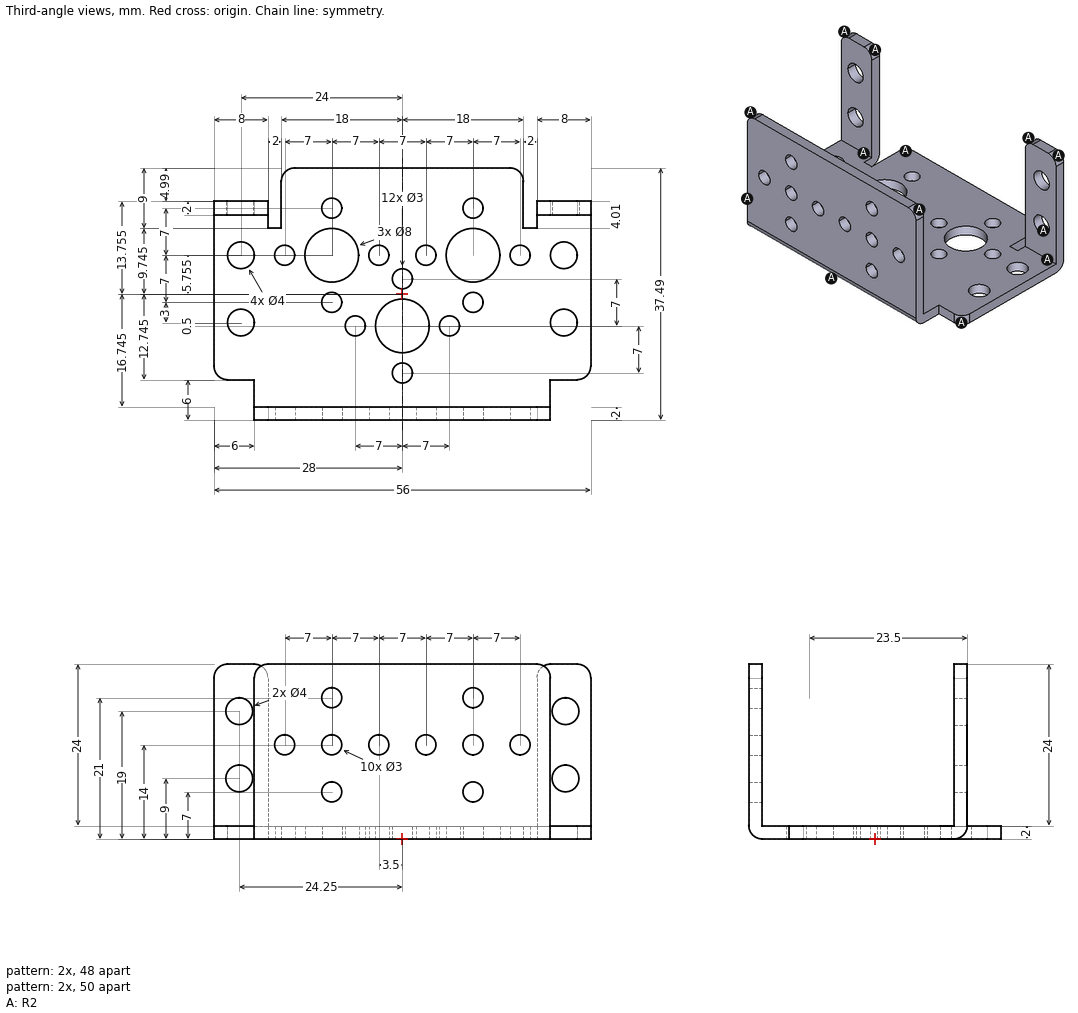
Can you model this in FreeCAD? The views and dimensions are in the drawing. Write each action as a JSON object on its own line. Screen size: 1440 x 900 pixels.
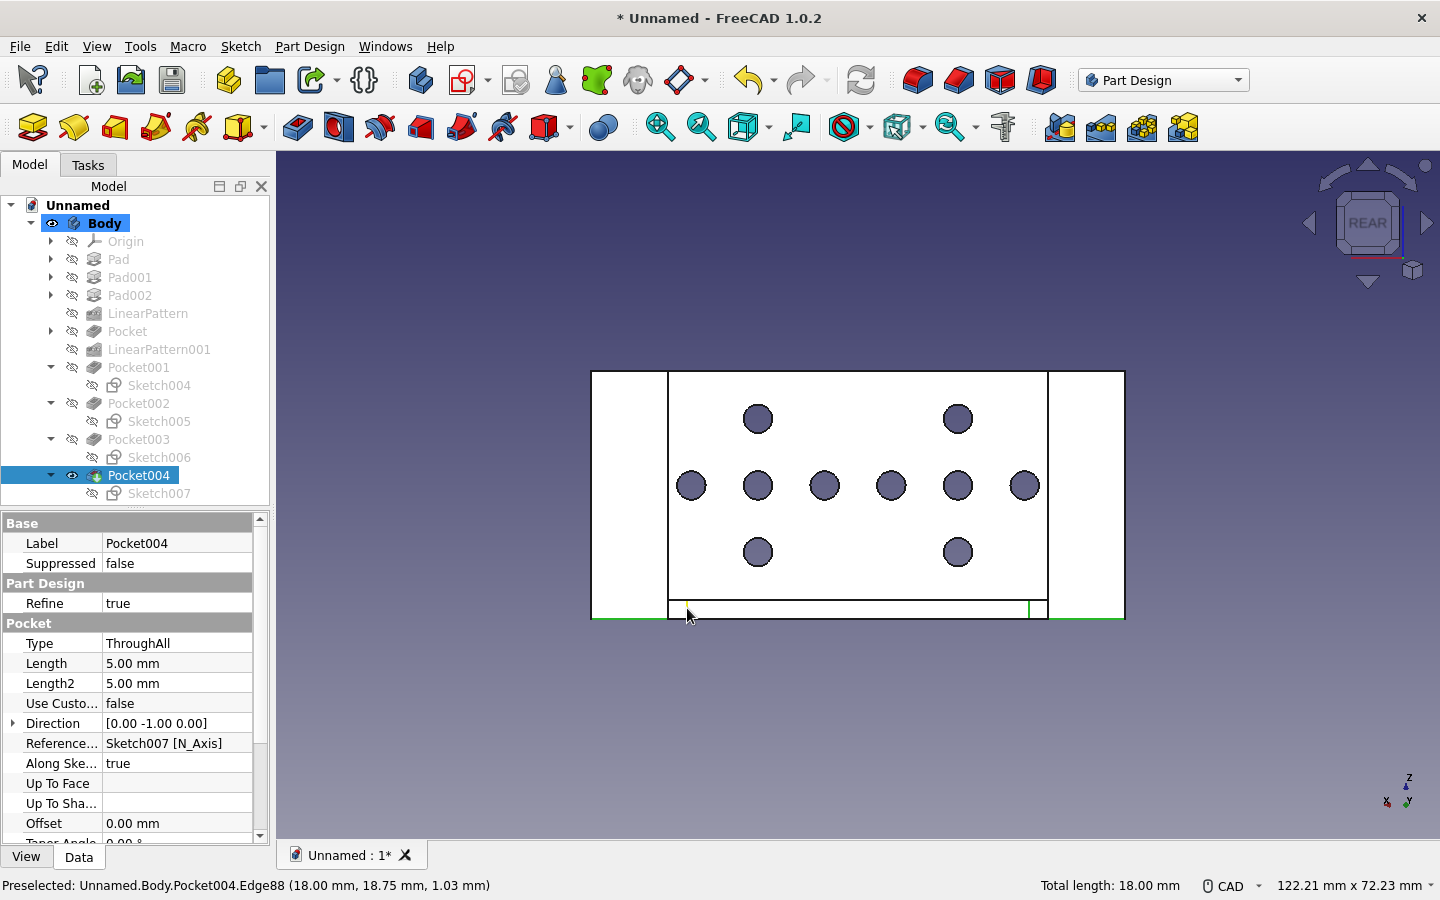
{"action": "key", "text": "0"}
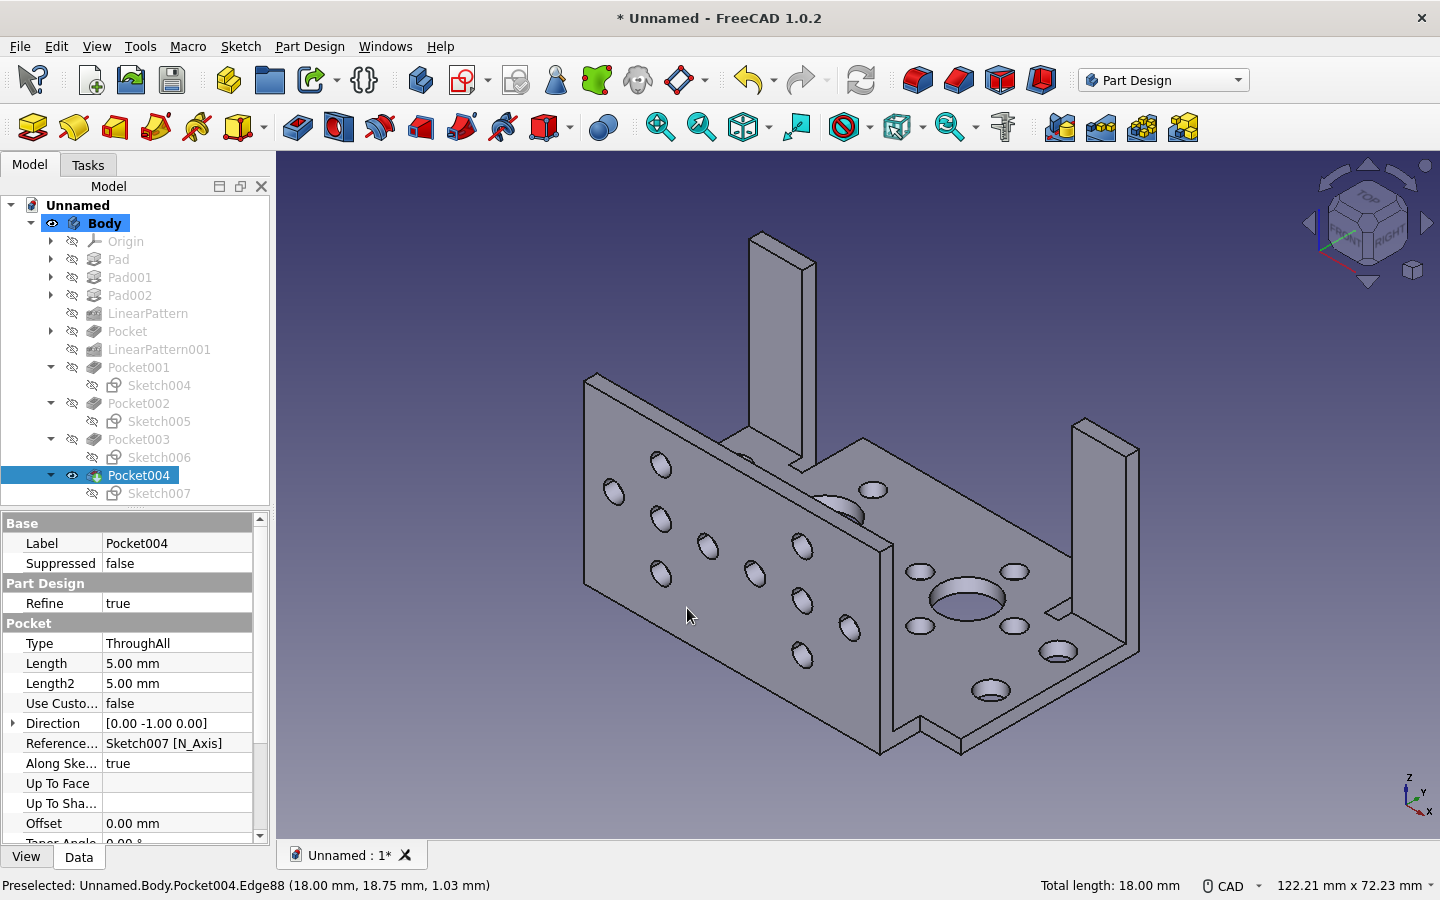
{"action": "left_click", "coordinate": [809, 266], "text": "ctrl"}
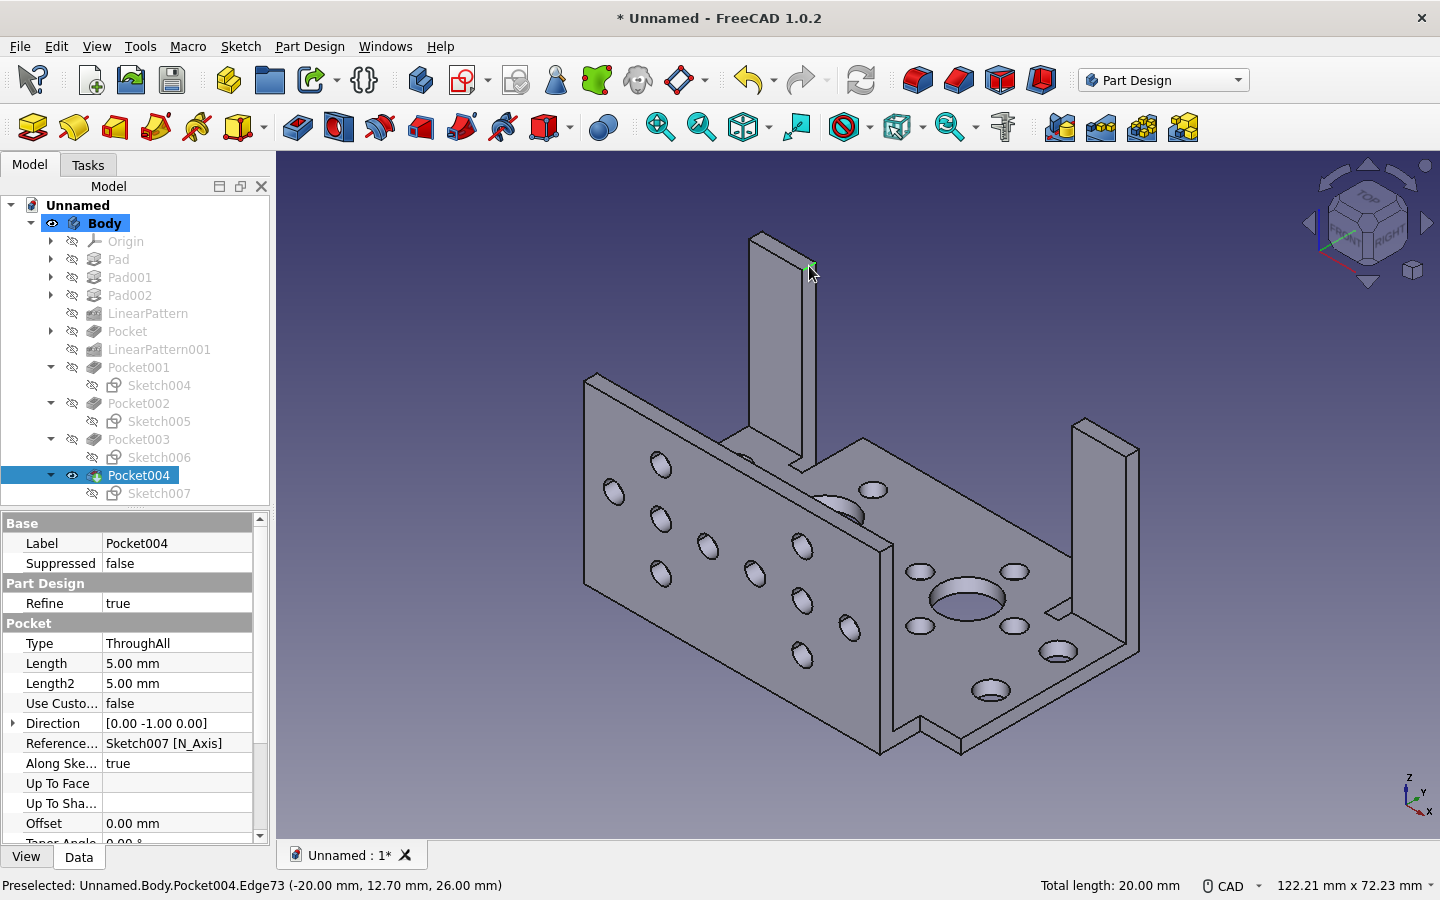
{"action": "left_click", "coordinate": [1132, 452], "text": "ctrl"}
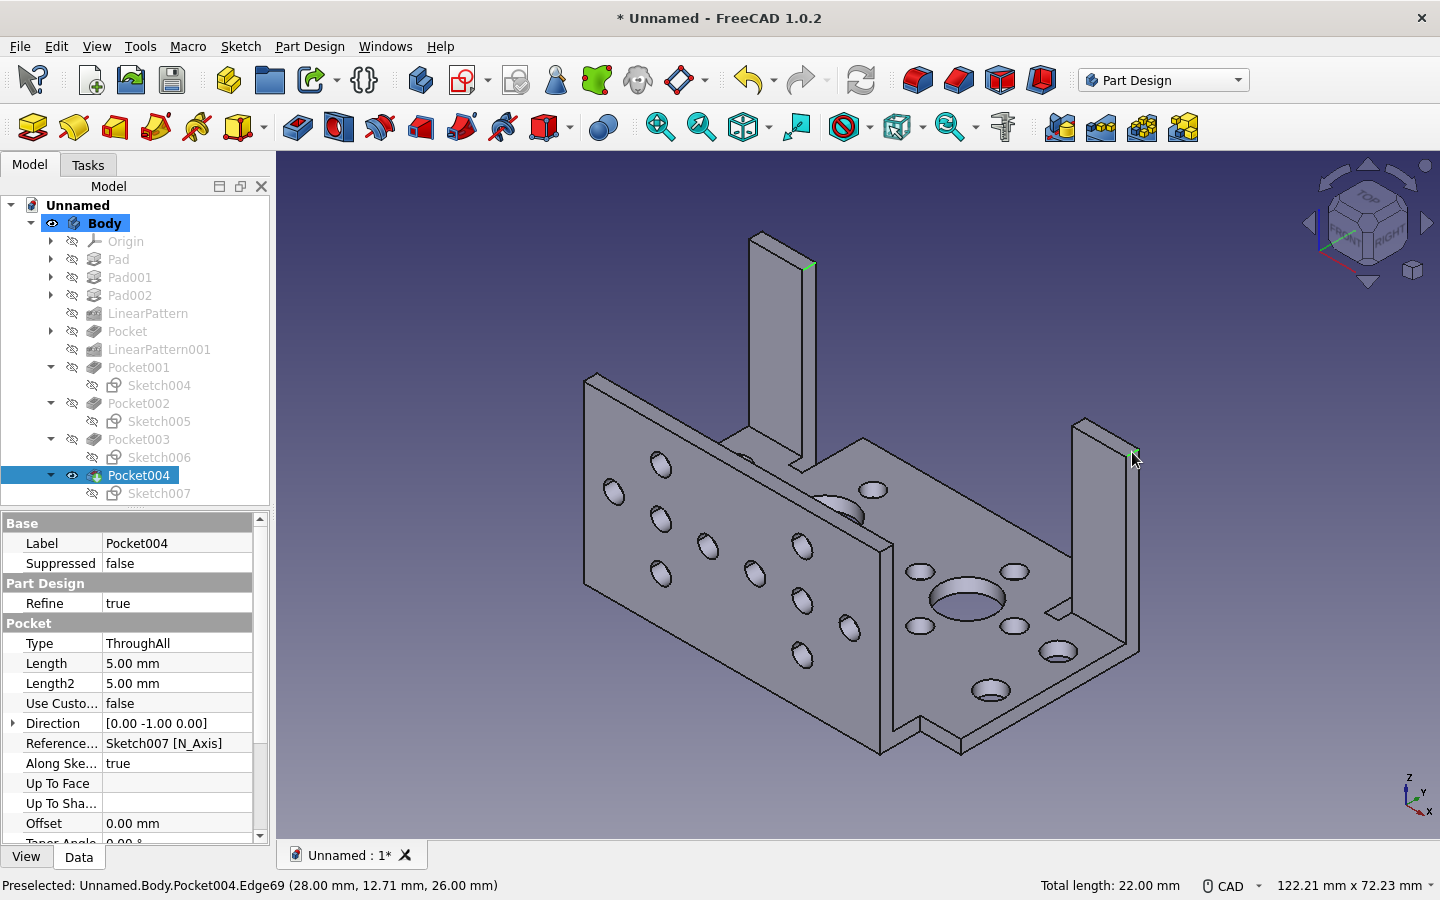
{"action": "left_click", "coordinate": [887, 547], "text": "ctrl"}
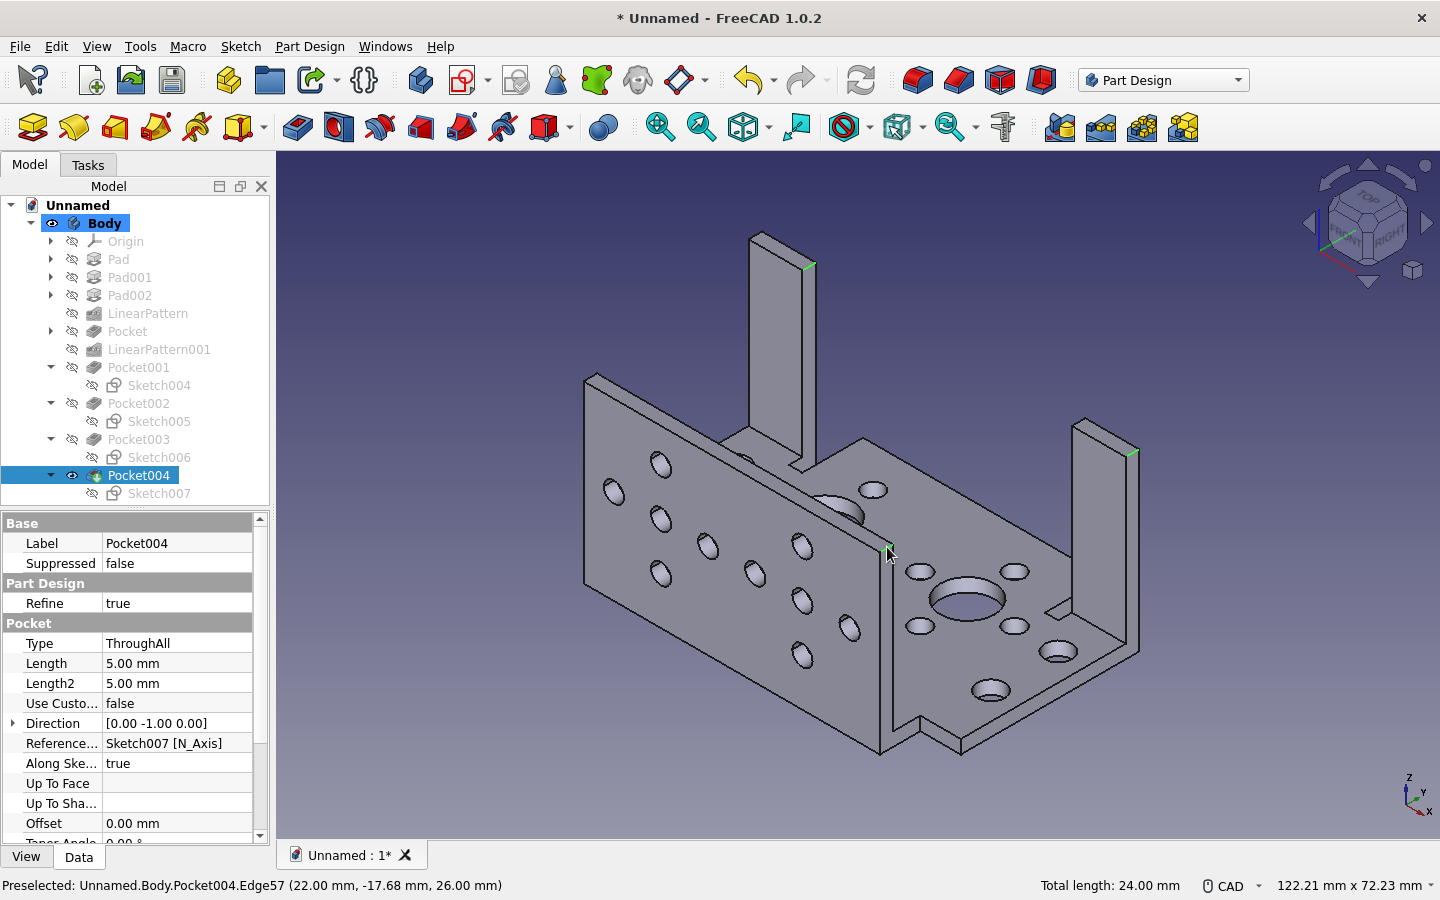
{"action": "left_click", "coordinate": [961, 746], "text": "ctrl"}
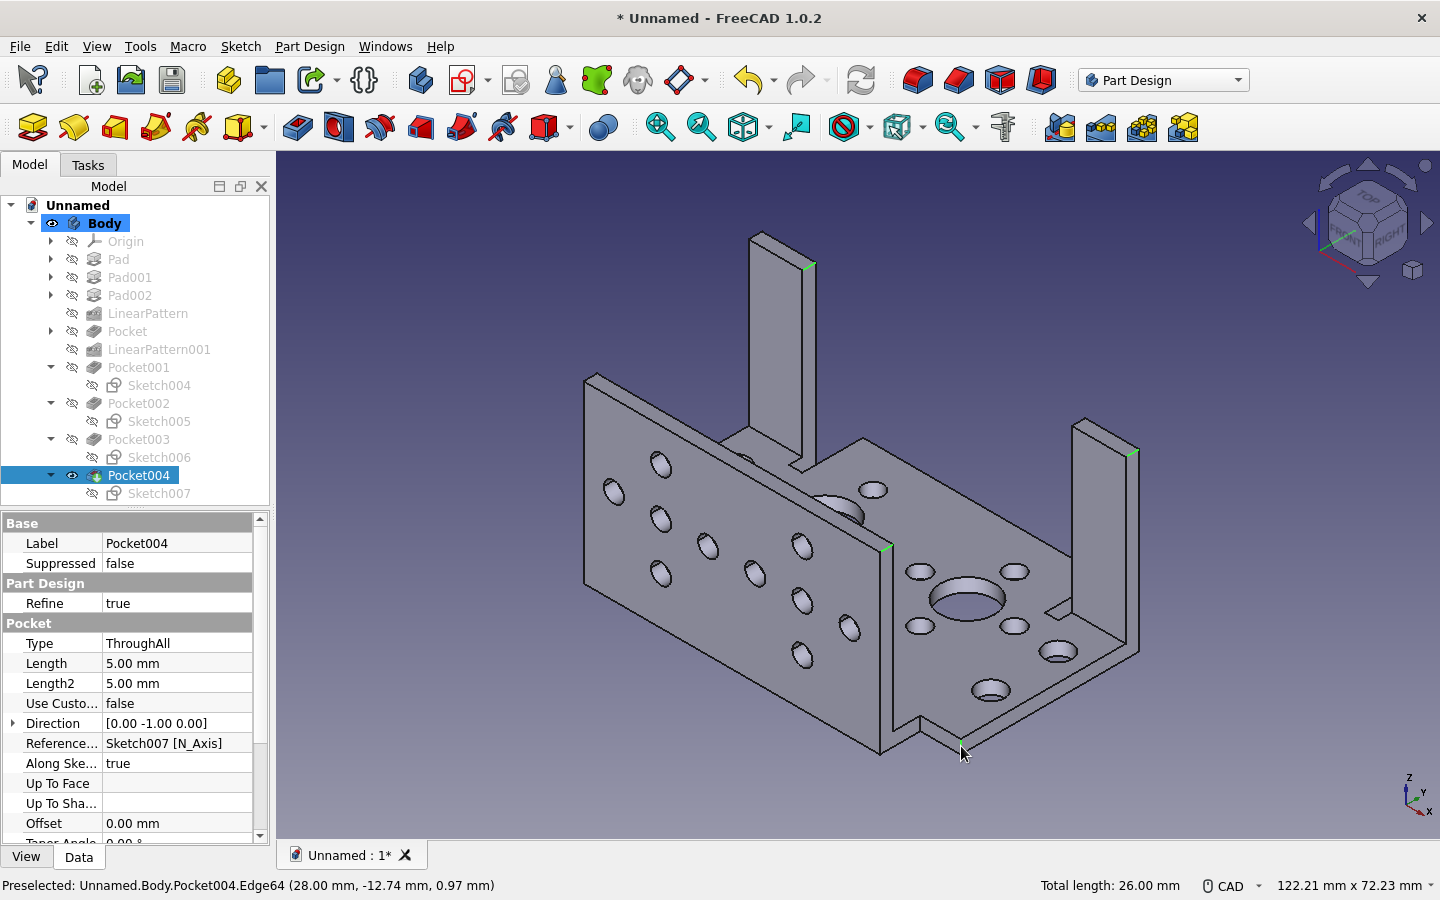
{"action": "scroll", "coordinate": [1105, 584], "scroll_direction": "up", "scroll_amount": 4}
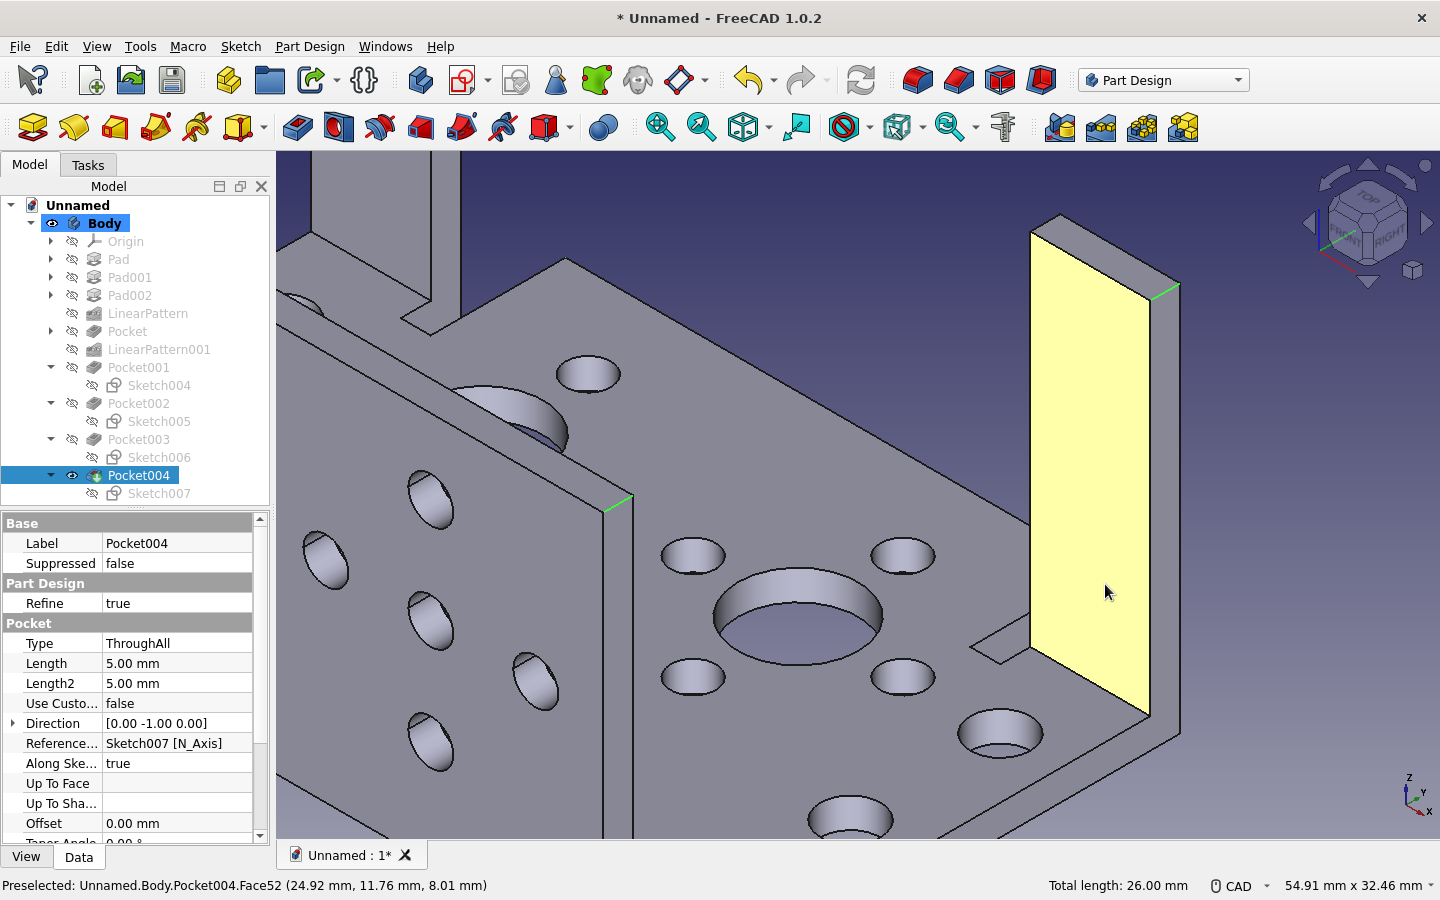
{"action": "key", "text": "v f"}